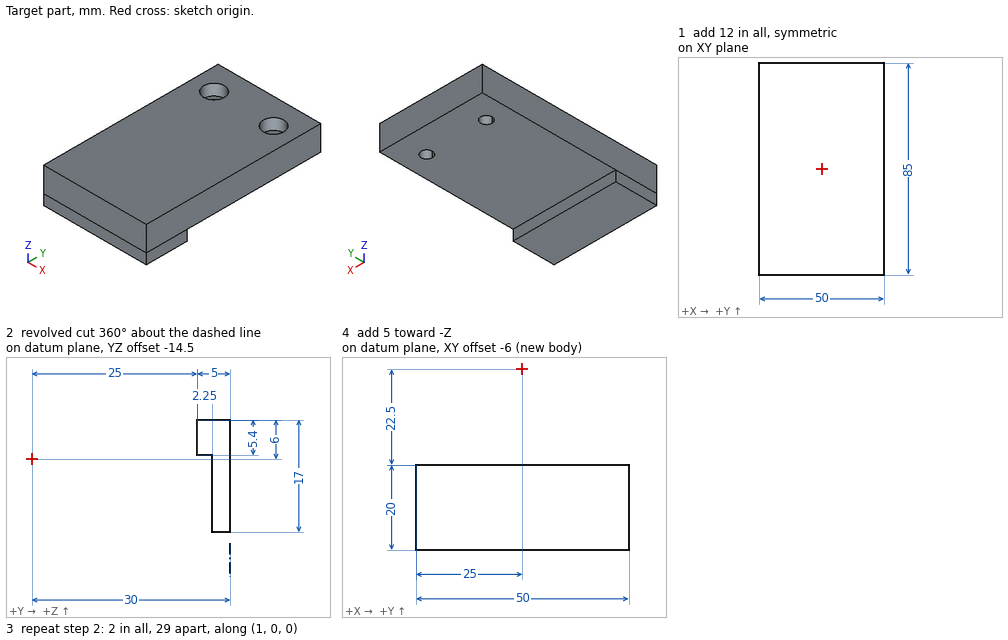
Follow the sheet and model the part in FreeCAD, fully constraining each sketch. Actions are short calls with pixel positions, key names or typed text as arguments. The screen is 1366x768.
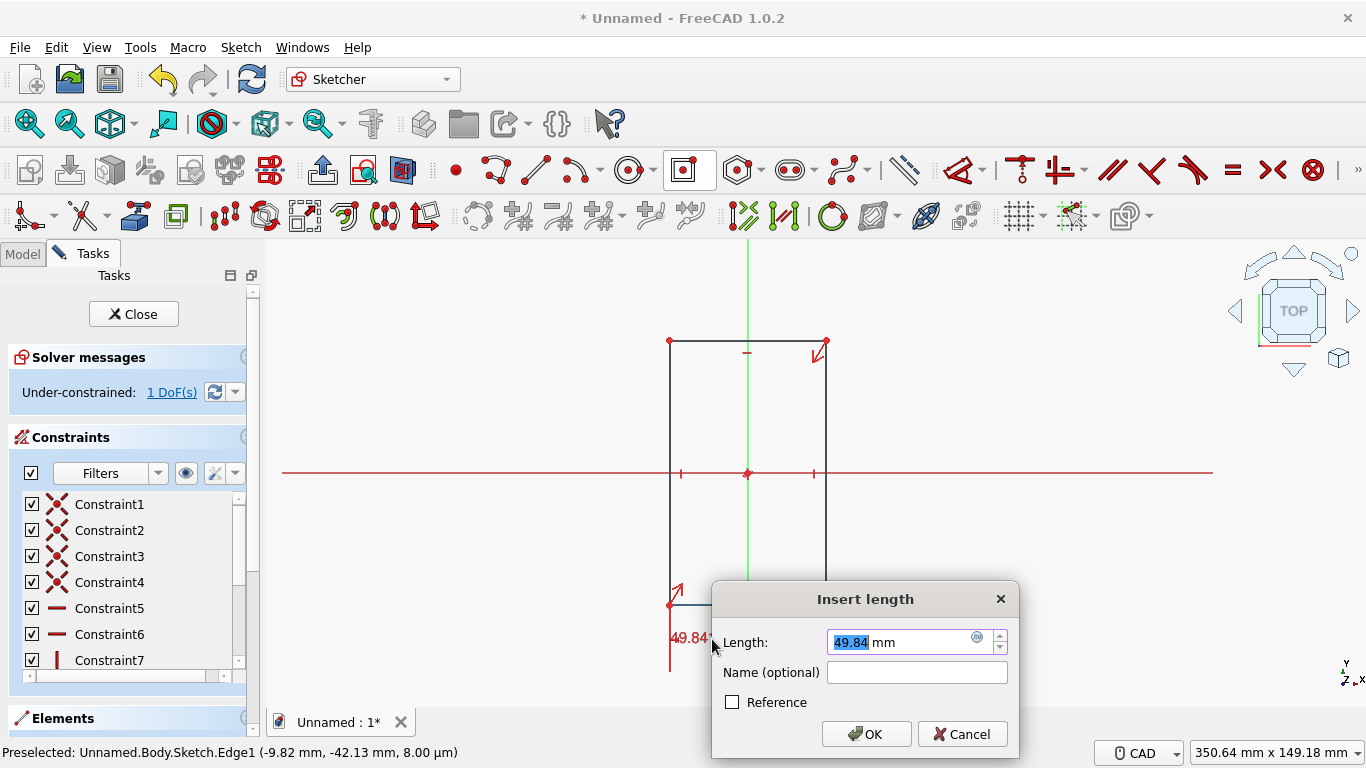
text(50)
key(Return)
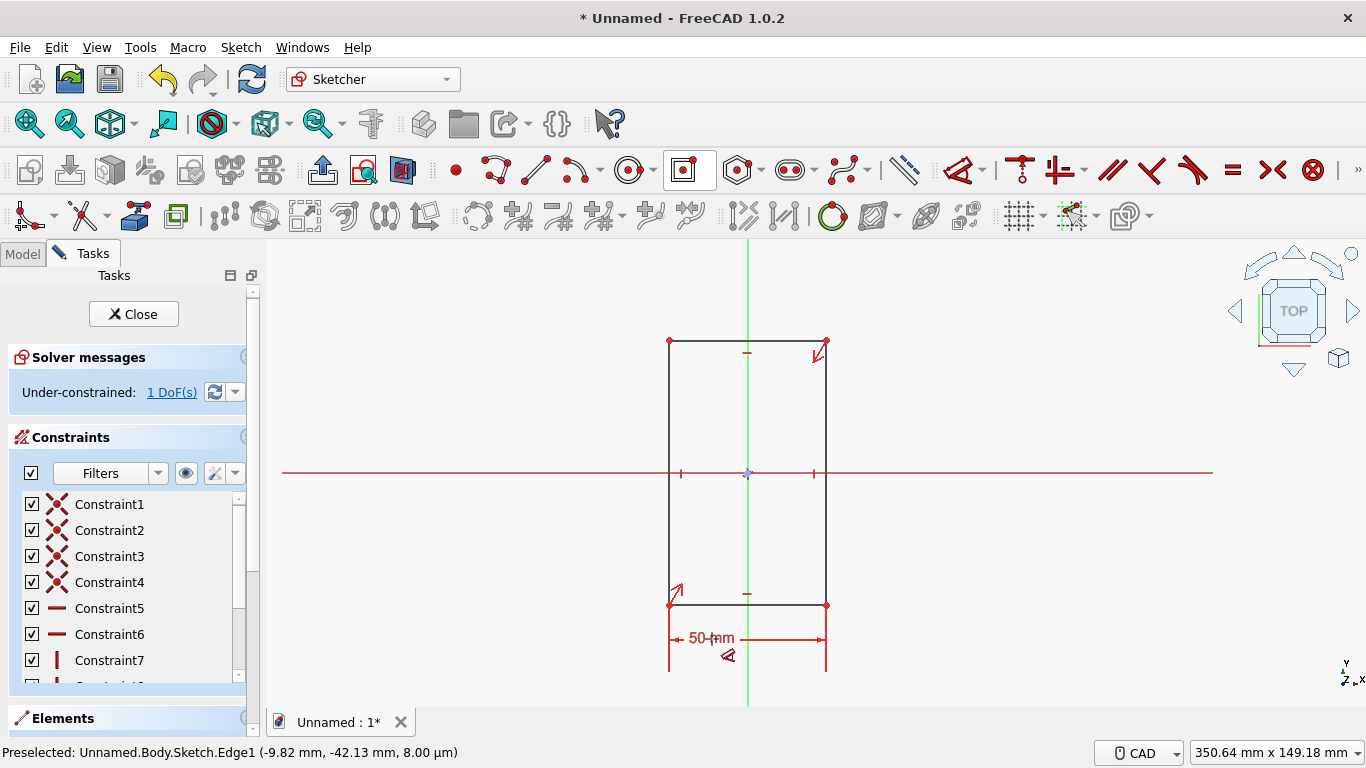
click(826, 526)
click(860, 412)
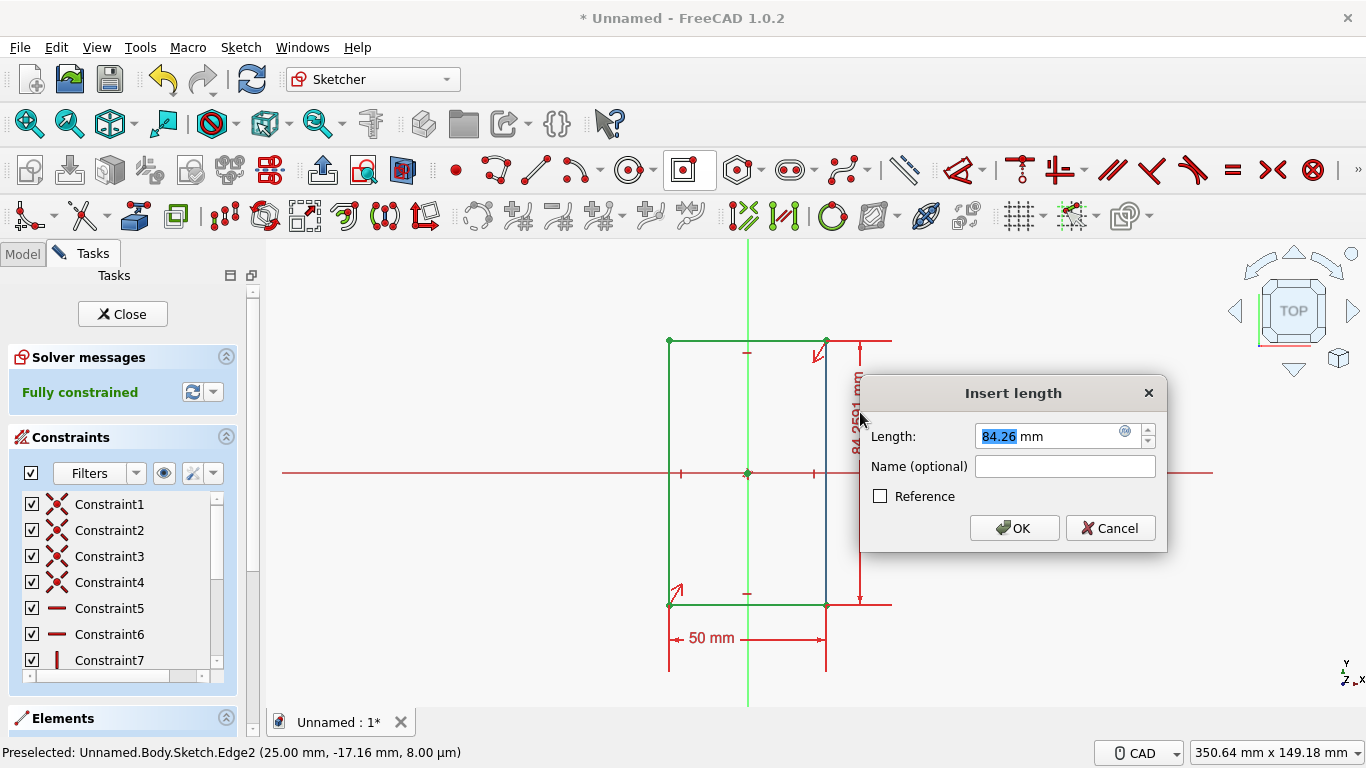
text(85)
key(Return)
key(Escape)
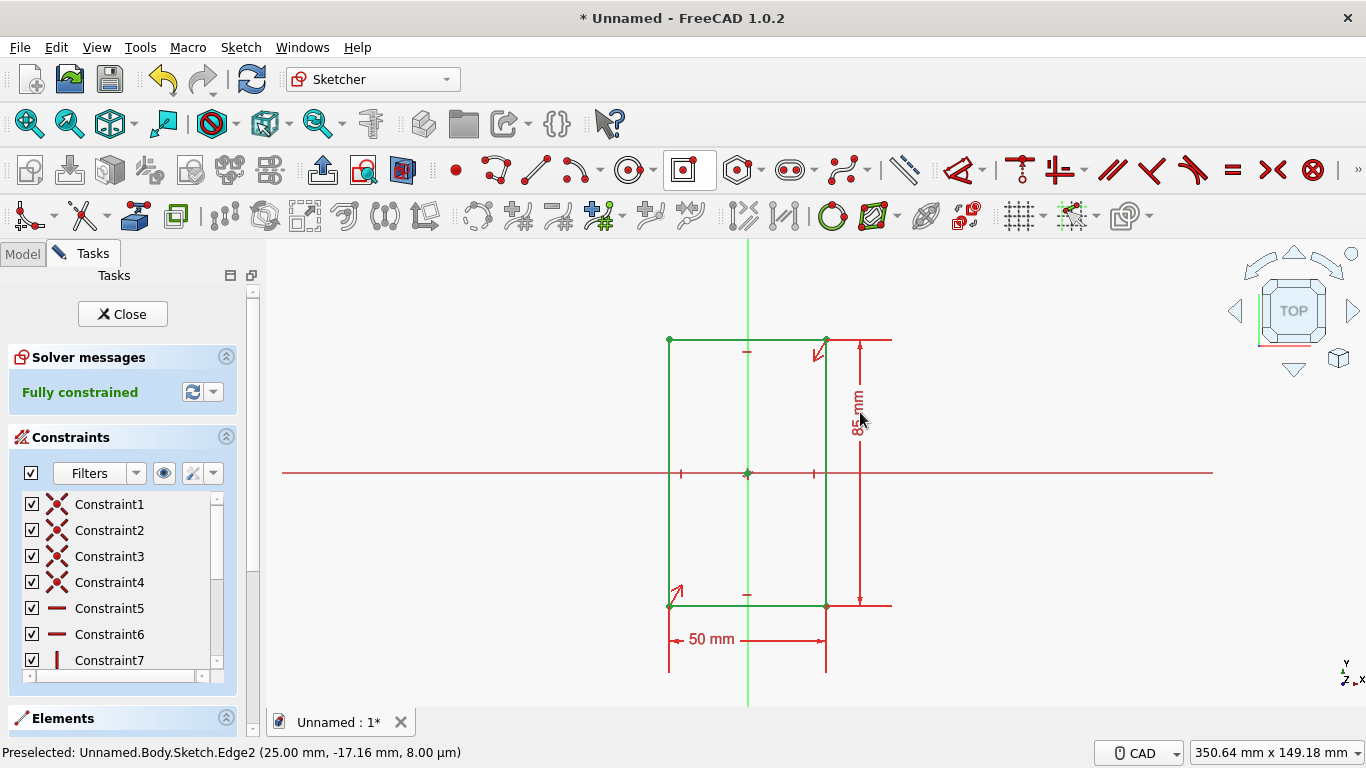
click(123, 314)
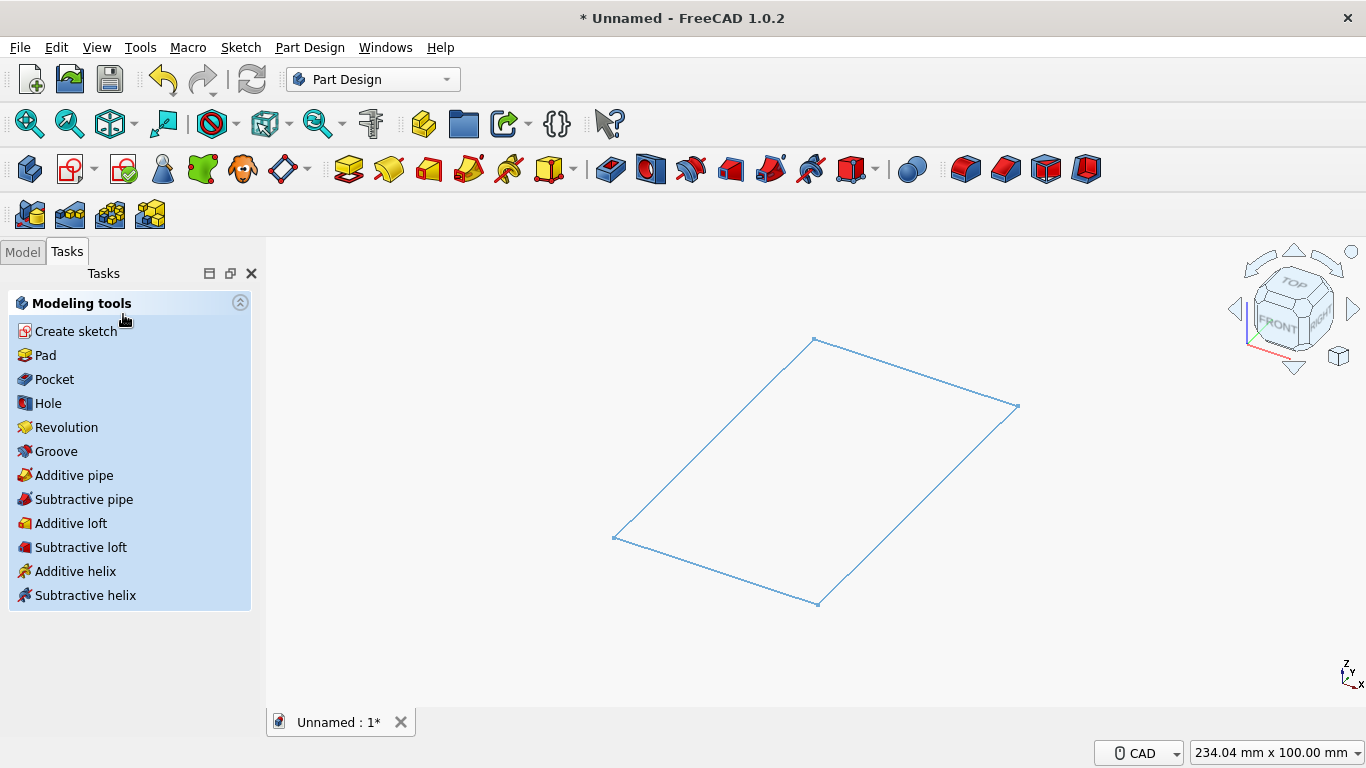
click(350, 170)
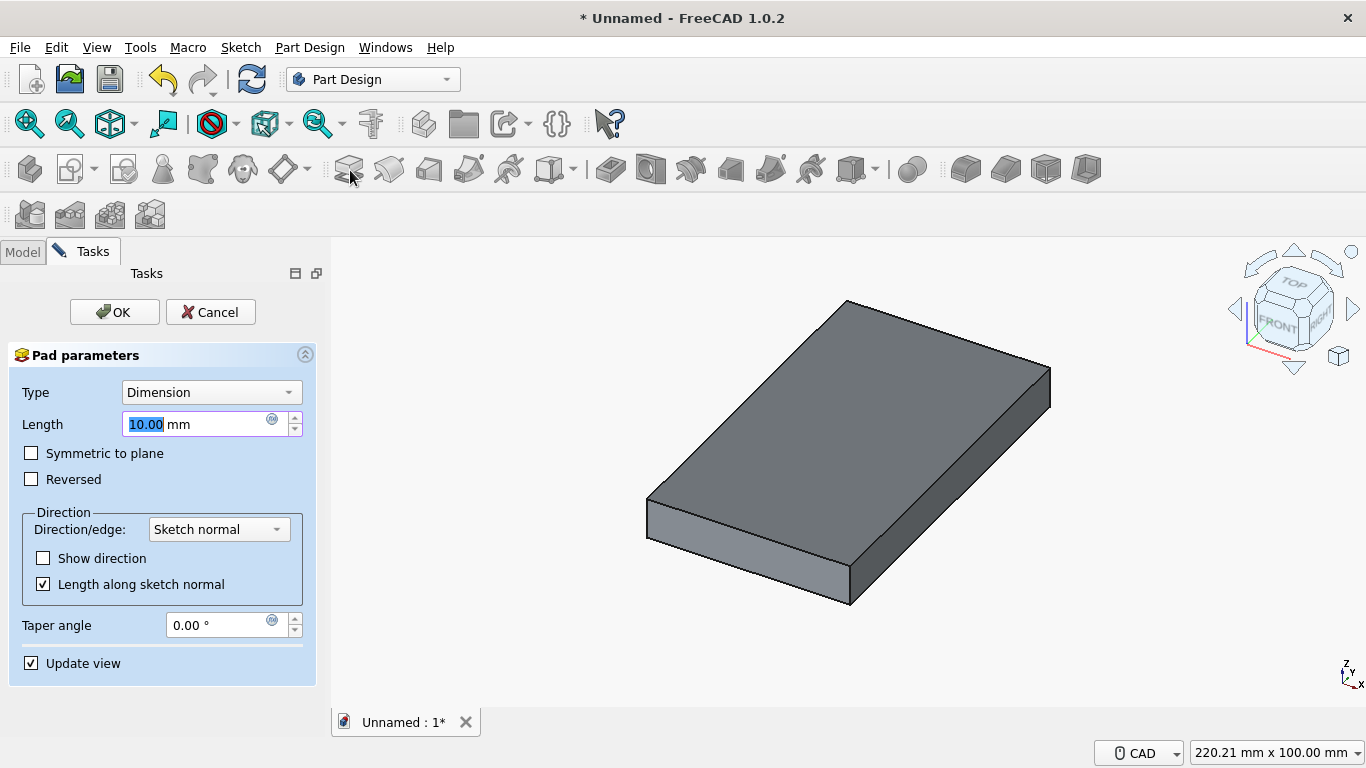
text(12)
key(Tab)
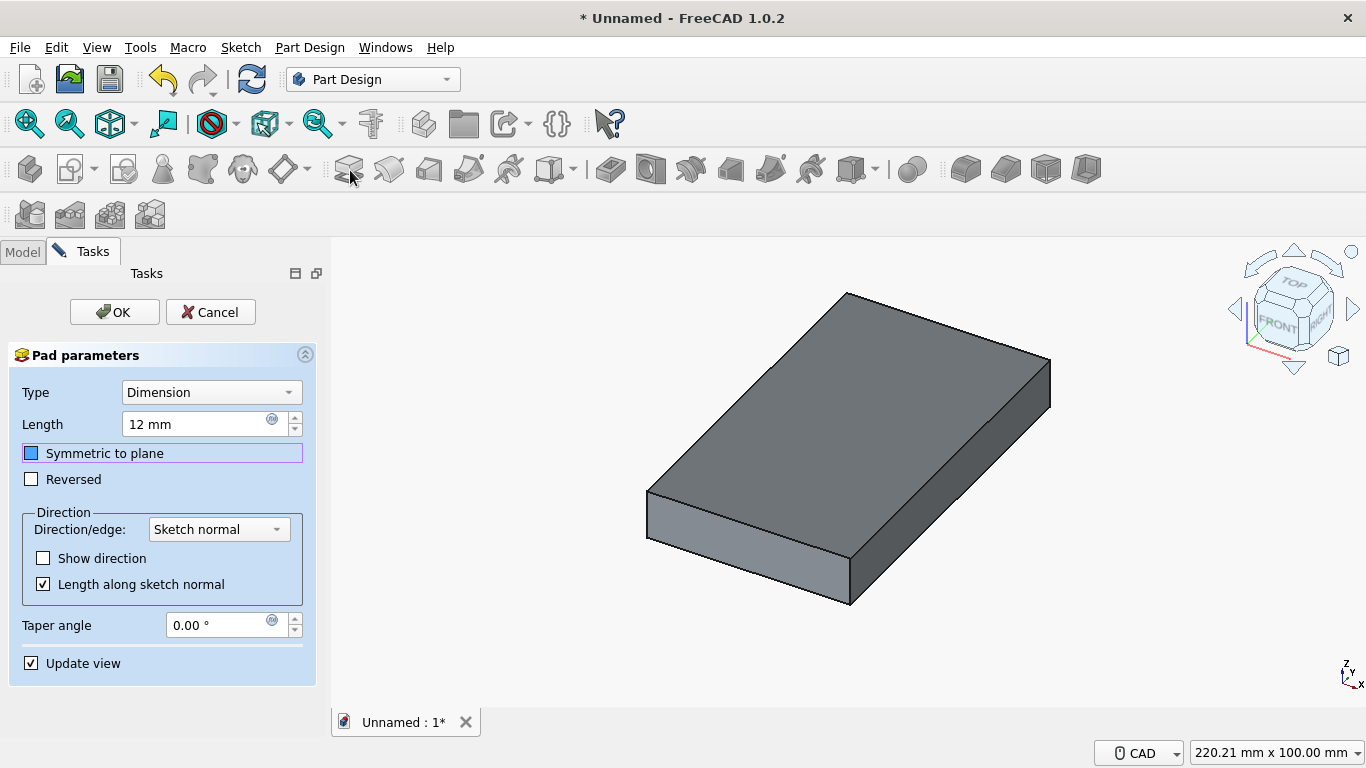
click(30, 453)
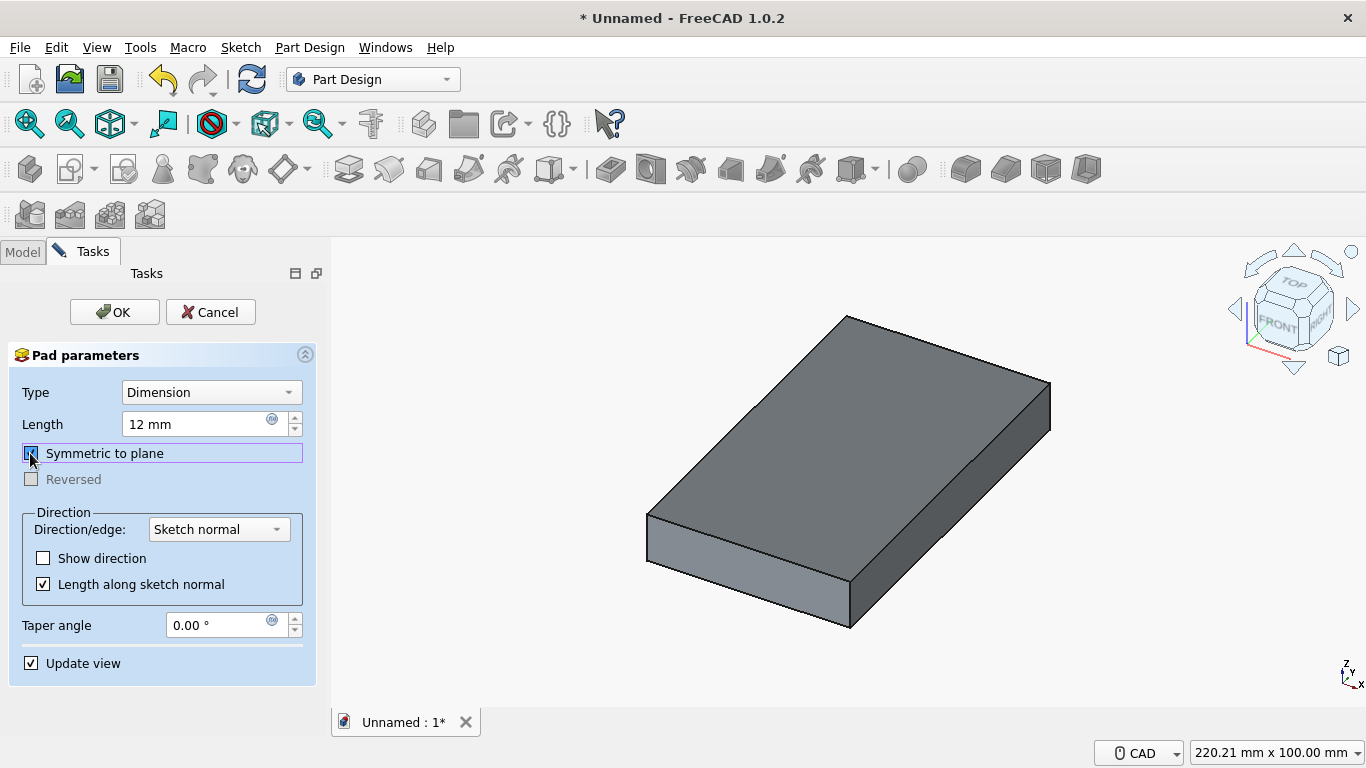
click(115, 312)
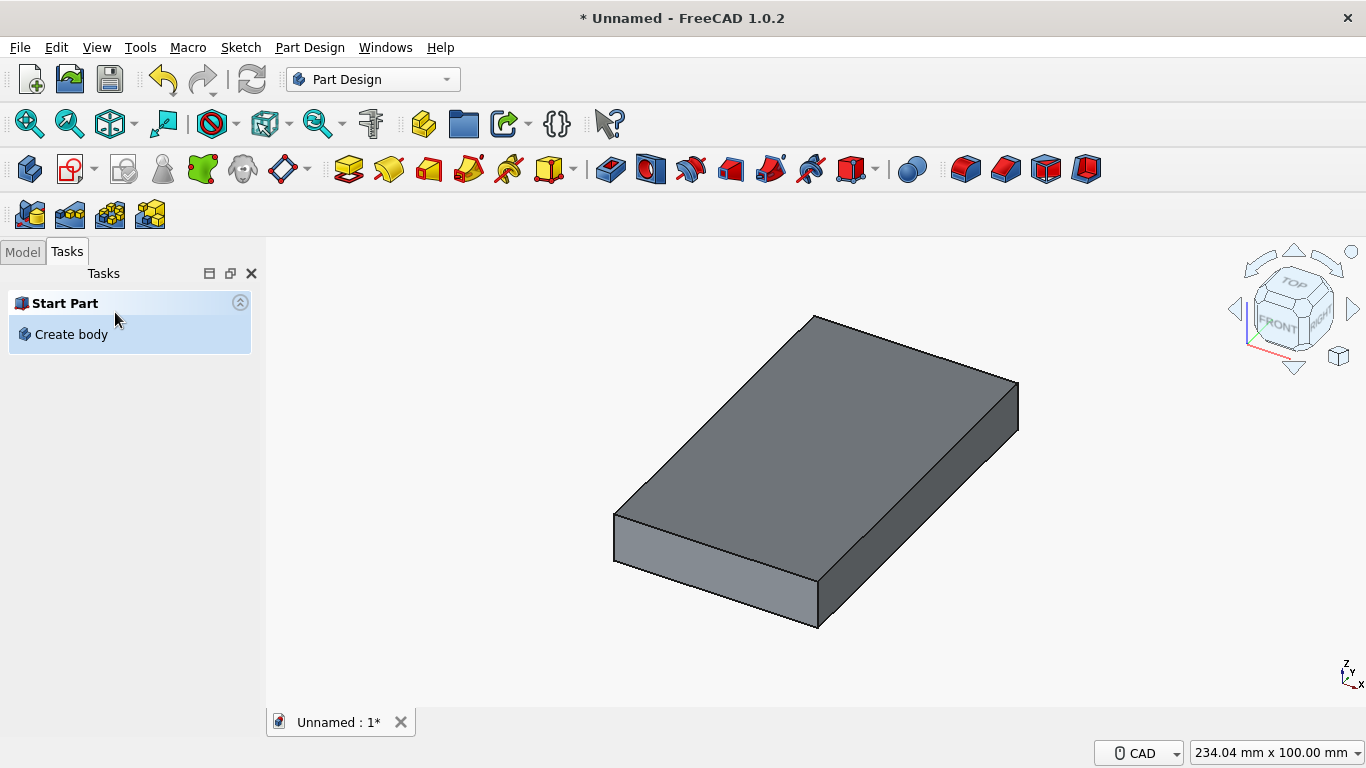
click(23, 251)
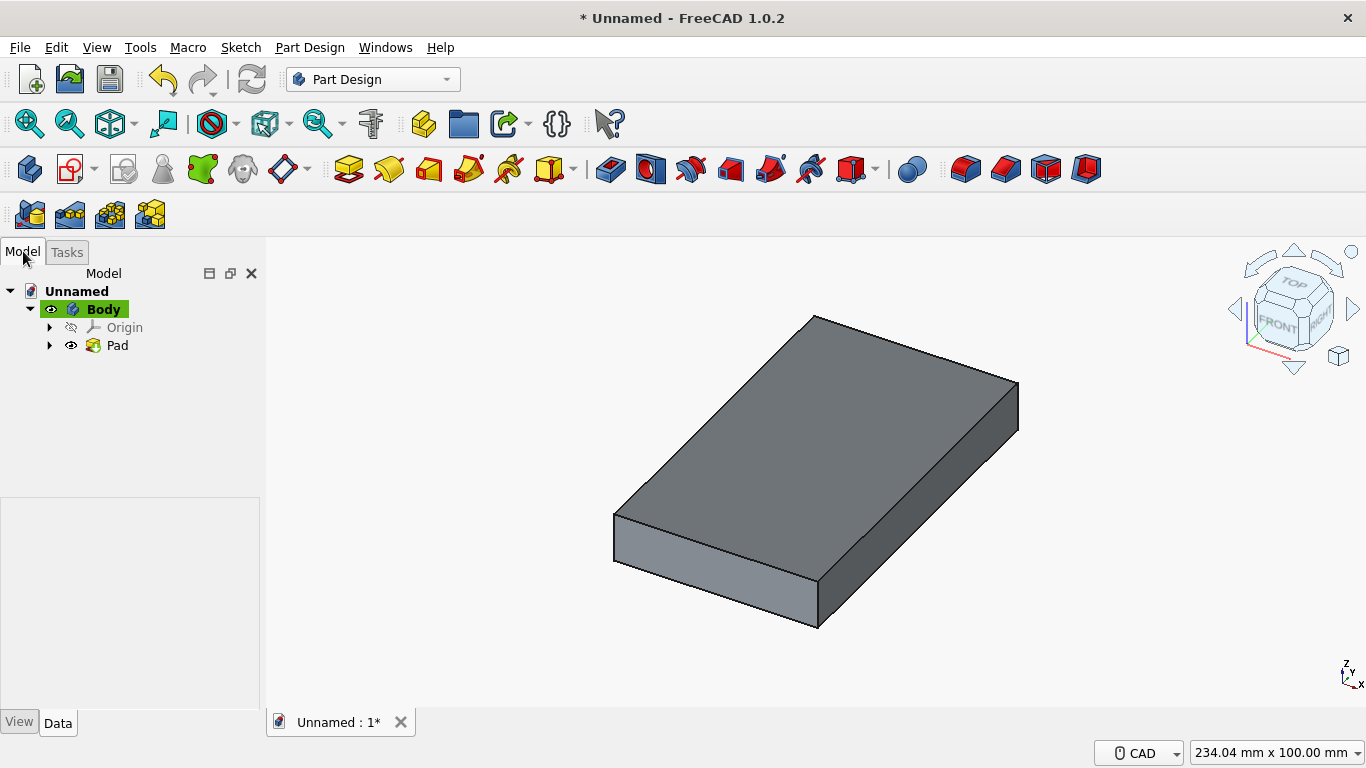
click(50, 327)